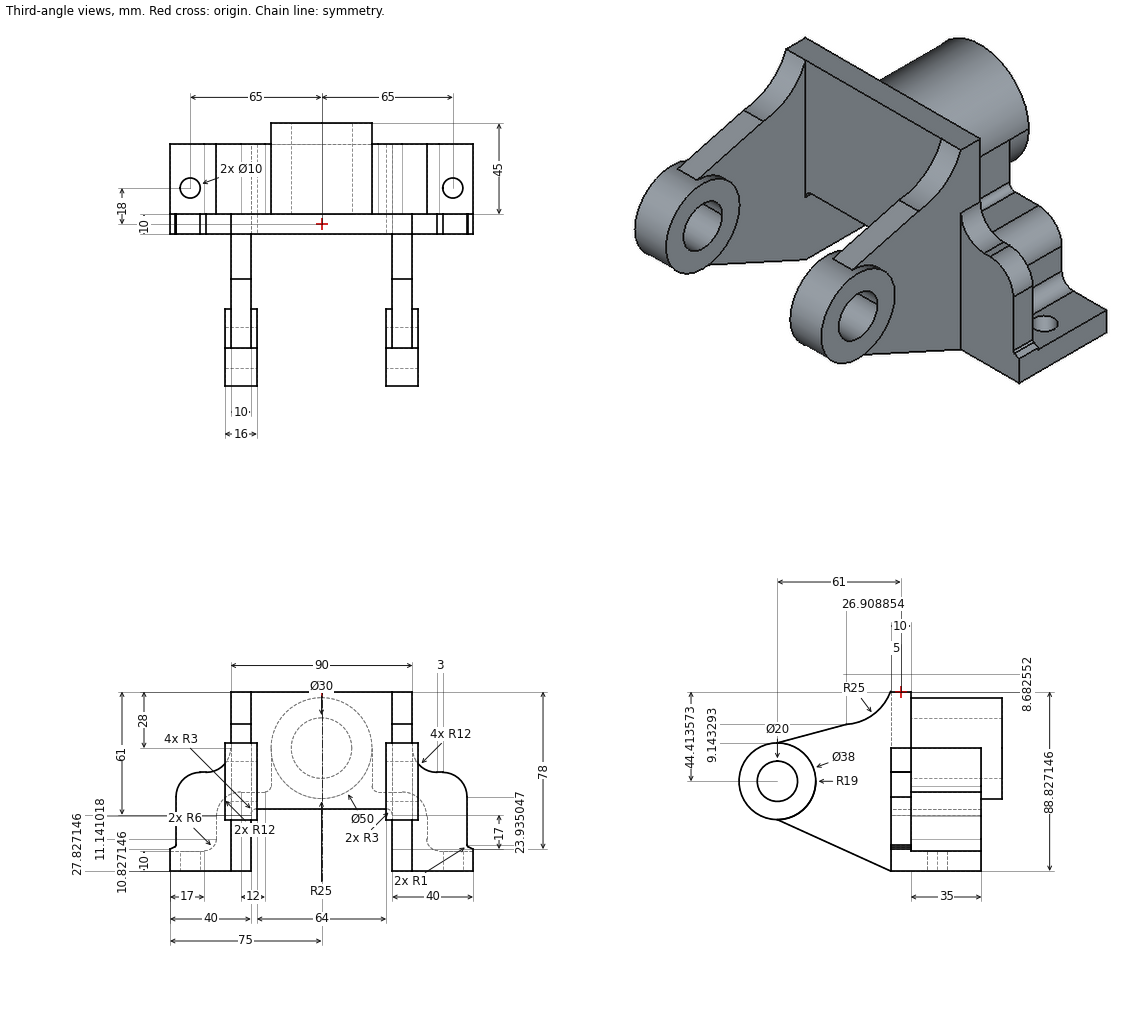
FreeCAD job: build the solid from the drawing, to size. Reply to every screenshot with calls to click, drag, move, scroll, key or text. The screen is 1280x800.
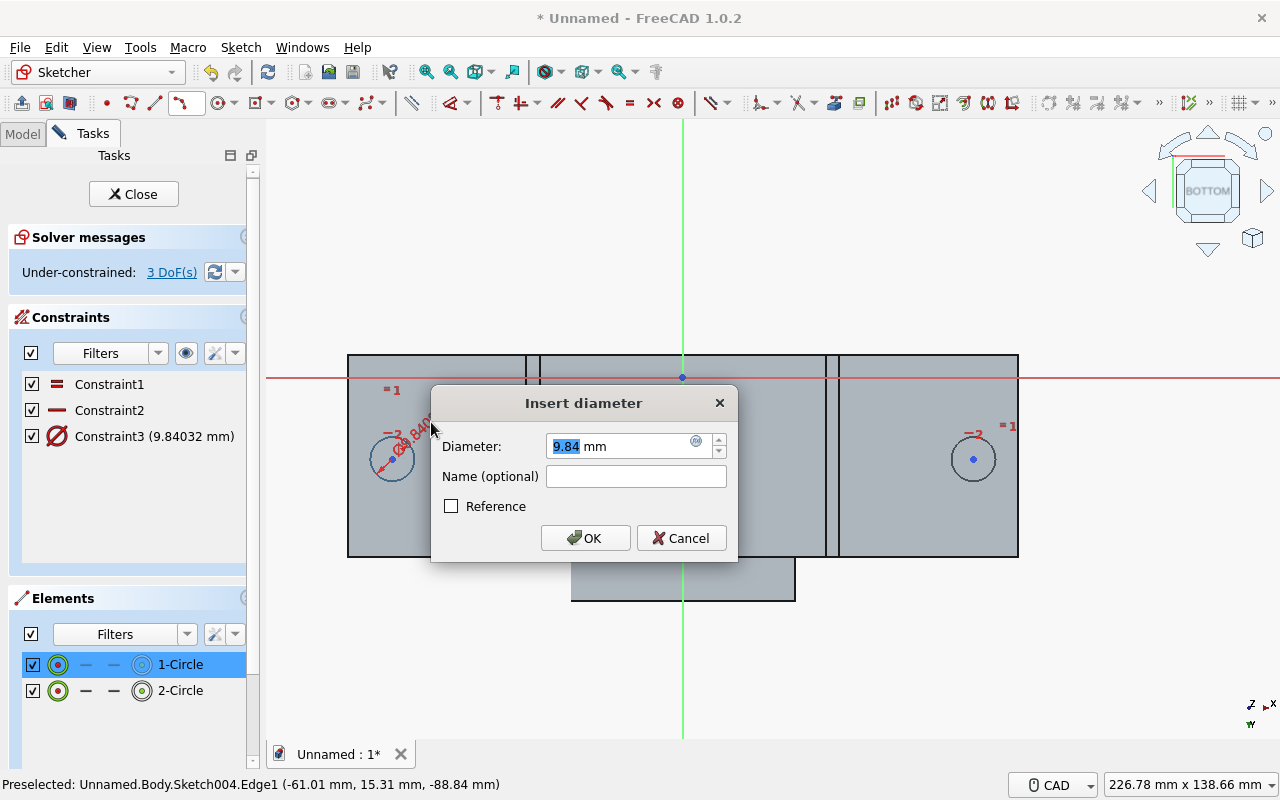
text(10)
key(Return)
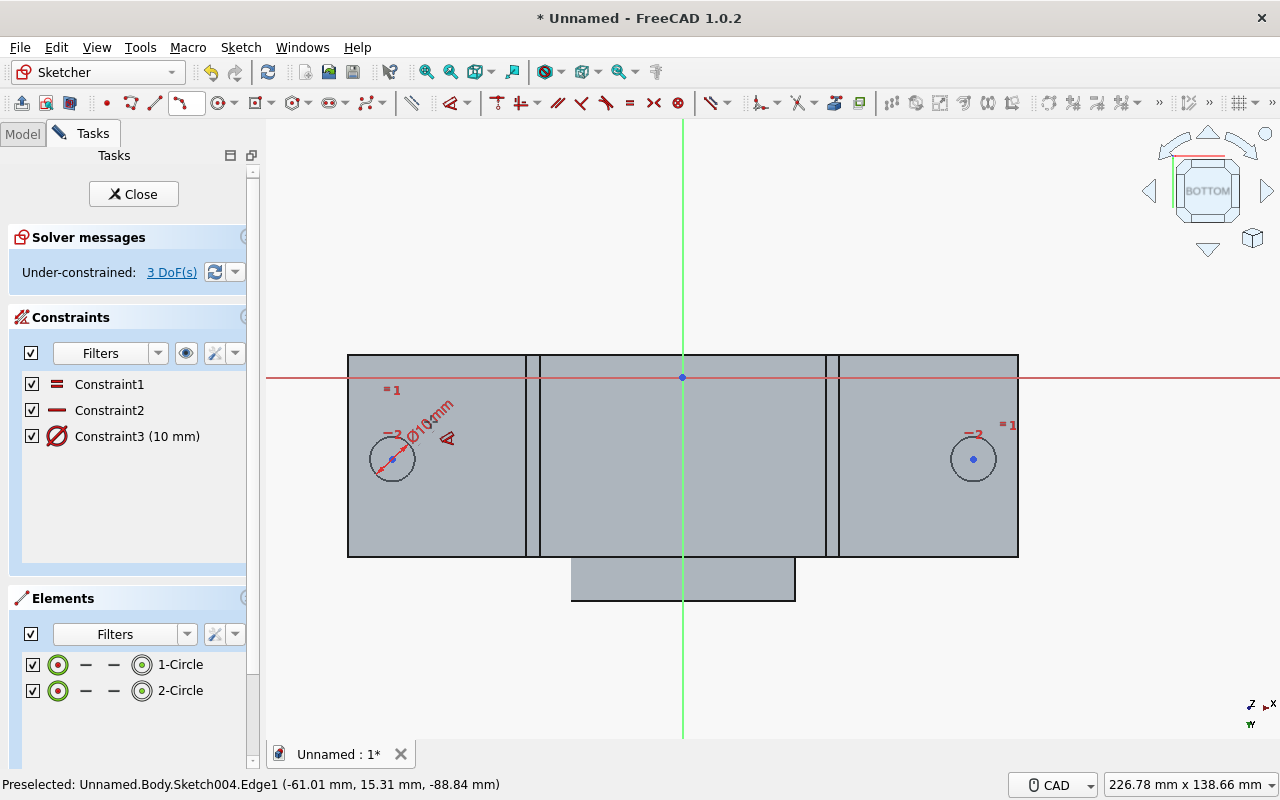
click(392, 459)
click(538, 344)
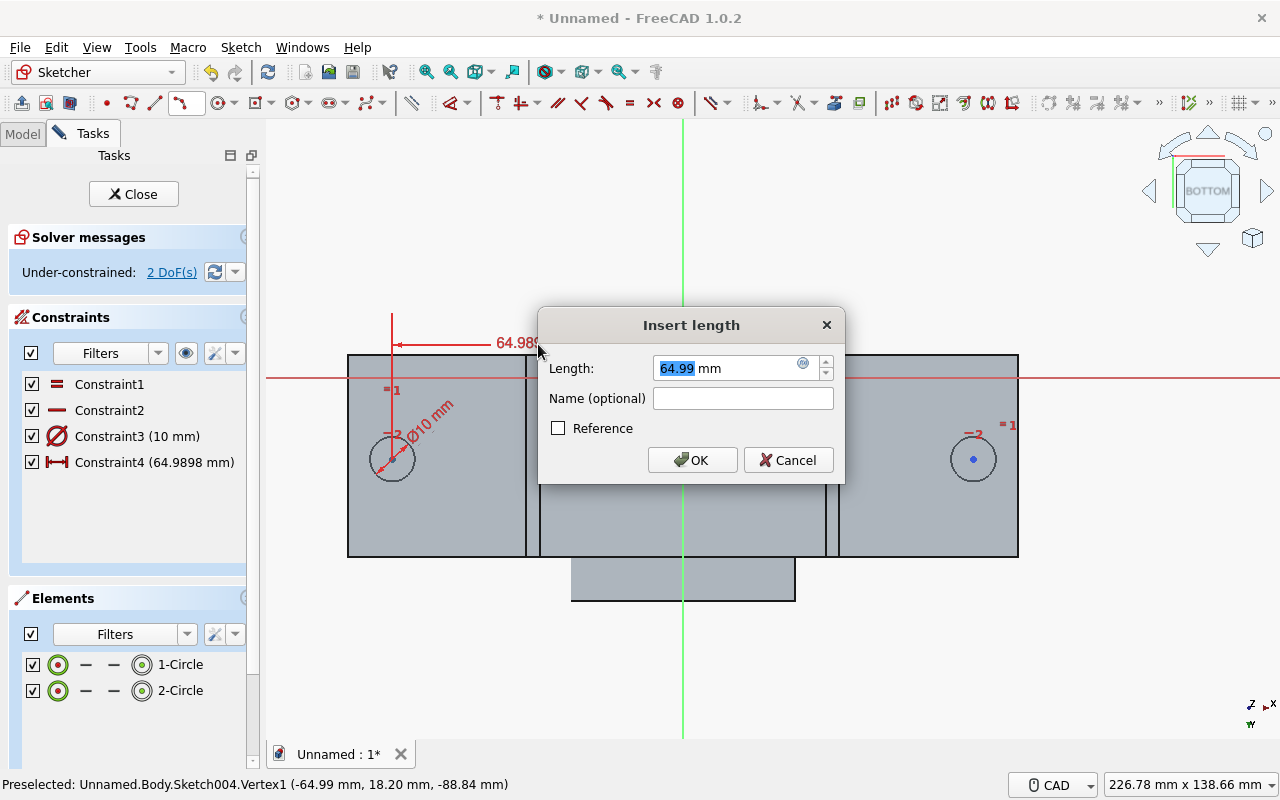
text(65)
key(Return)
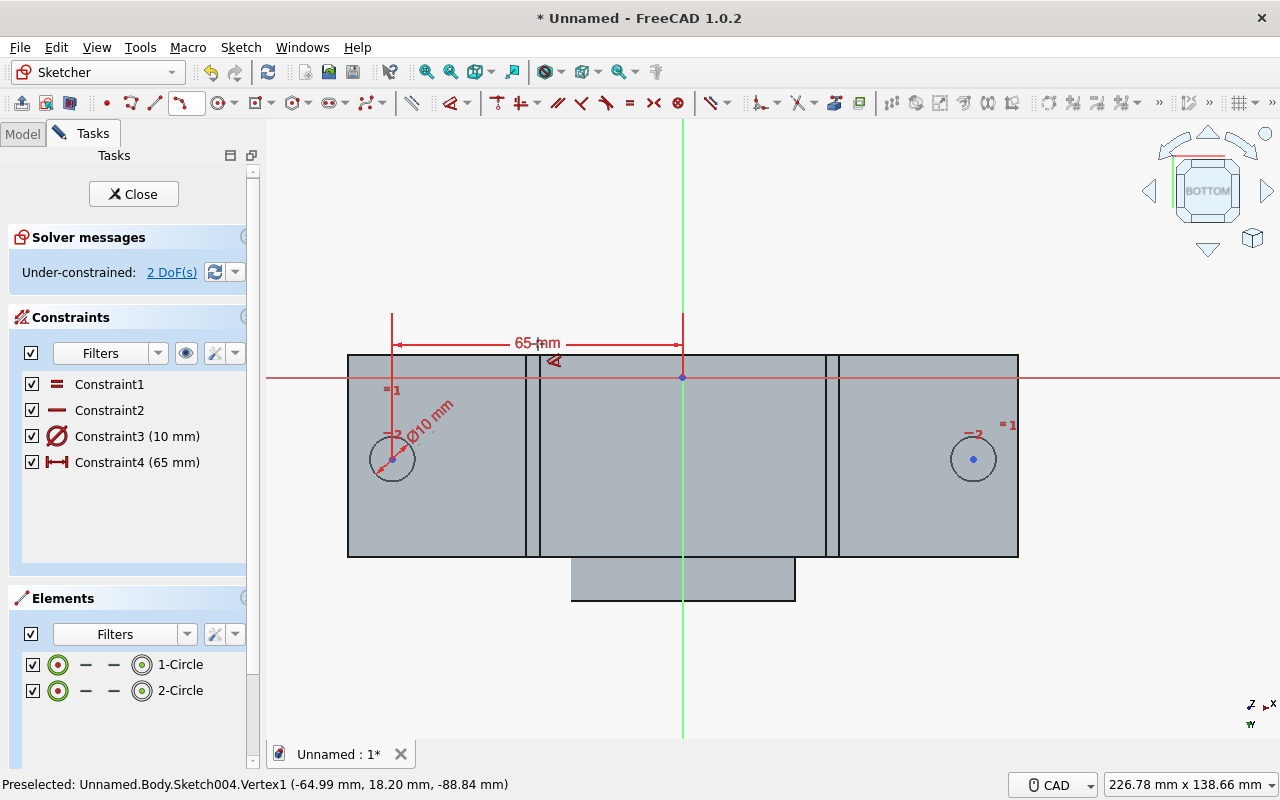
click(392, 459)
click(358, 418)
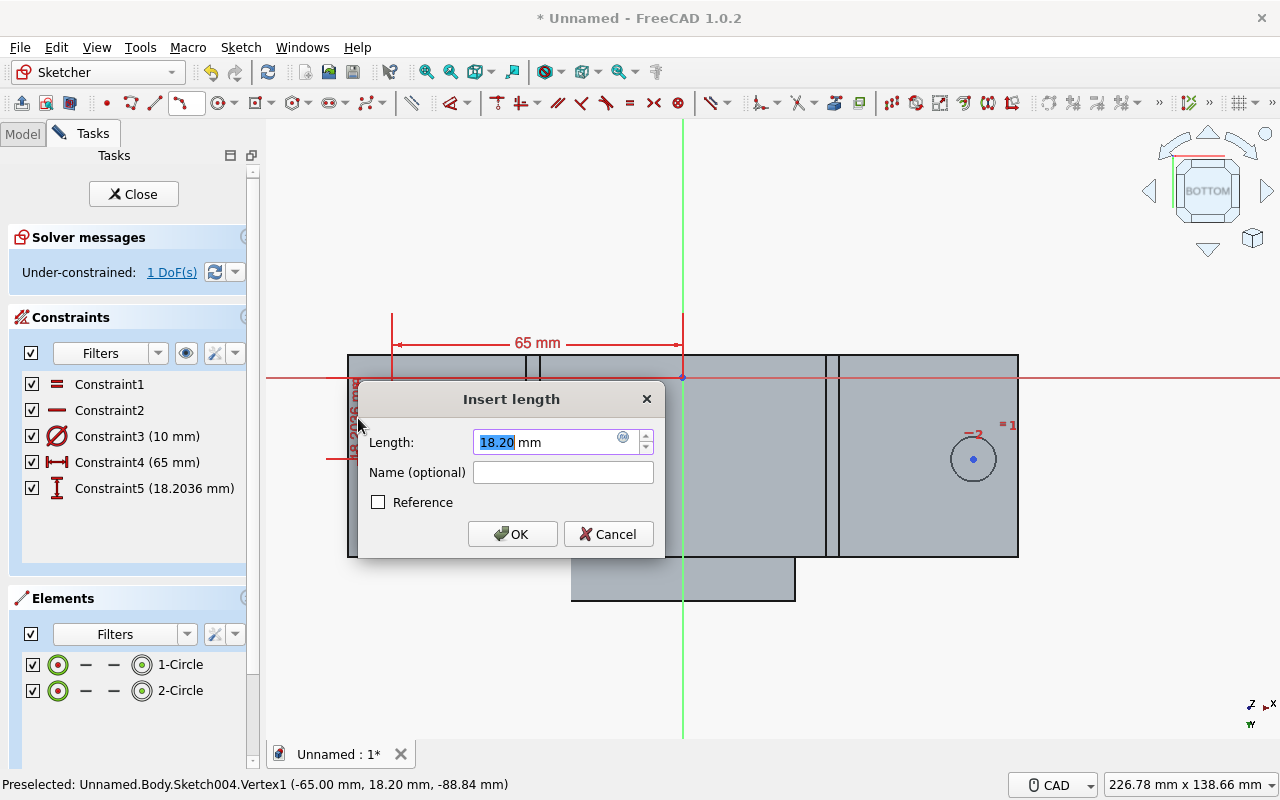
text(18)
key(Return)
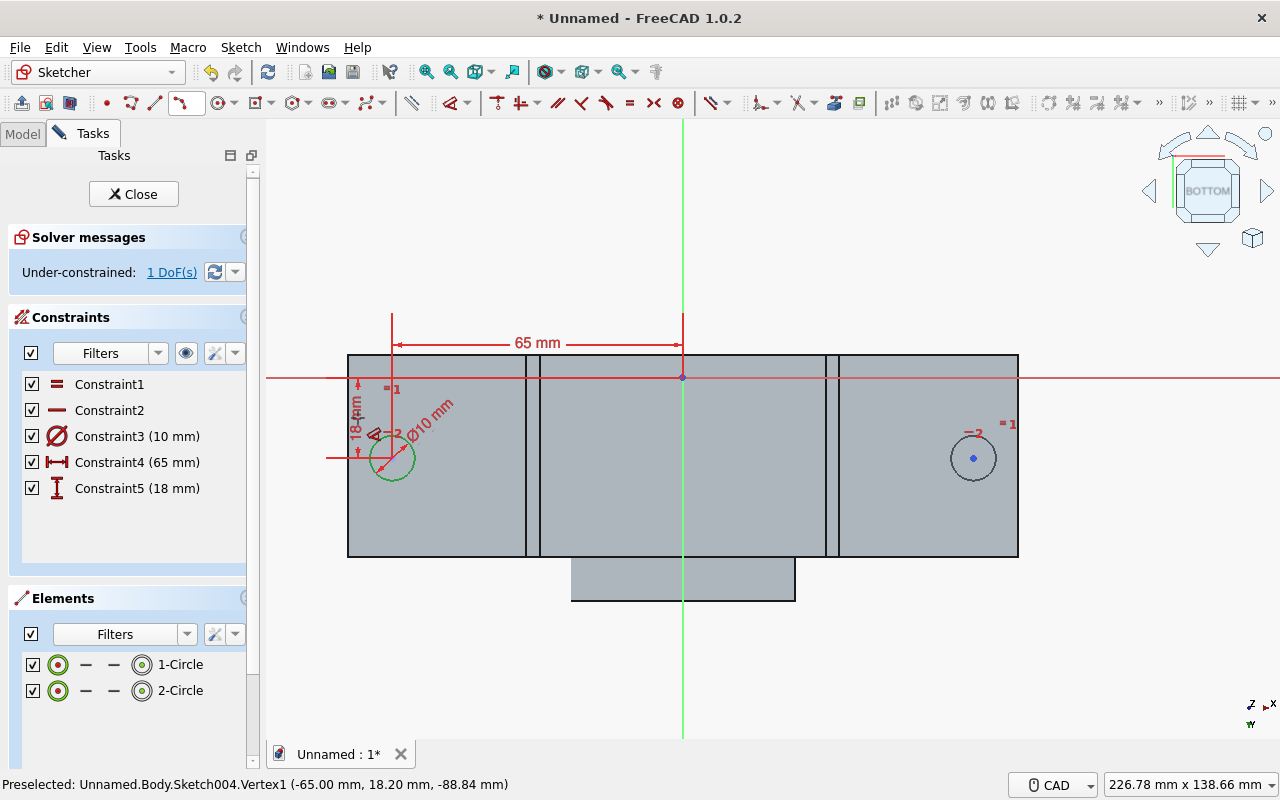
click(974, 458)
click(828, 344)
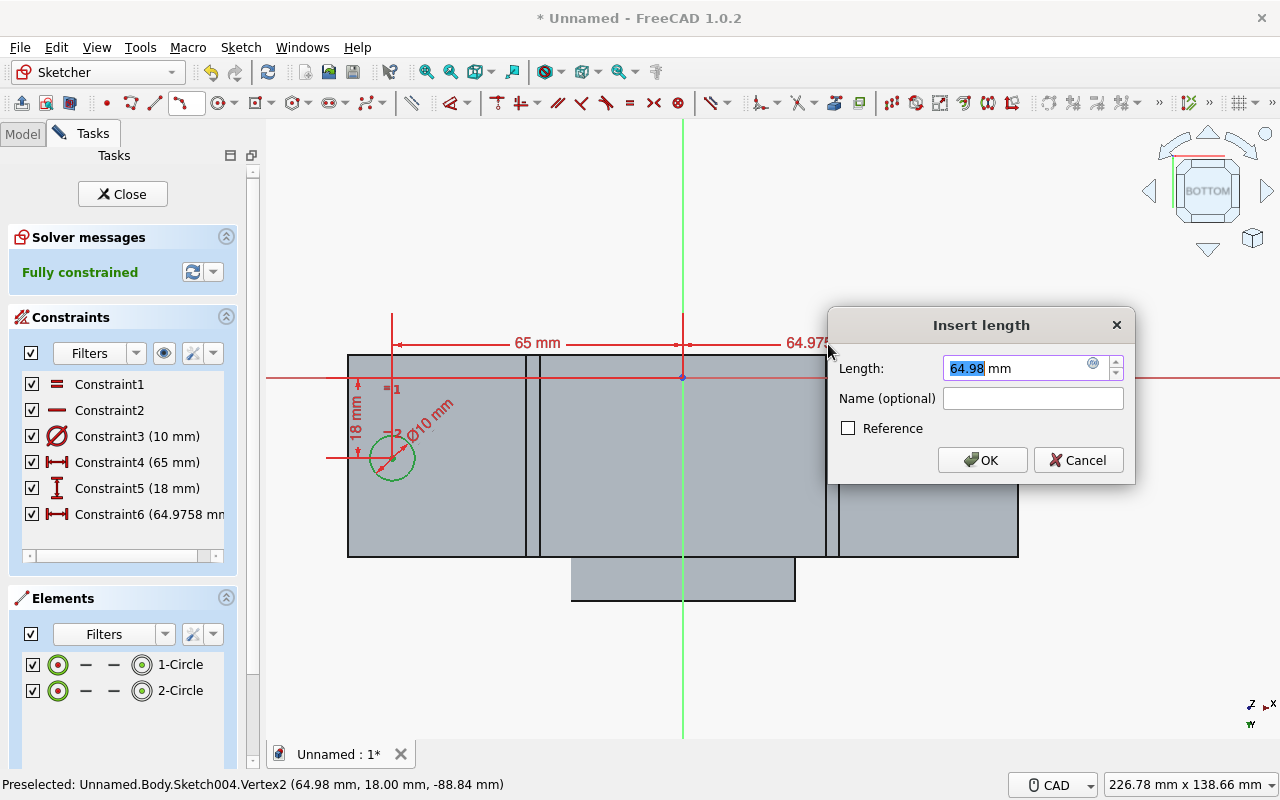
text(65)
key(Return)
key(Escape)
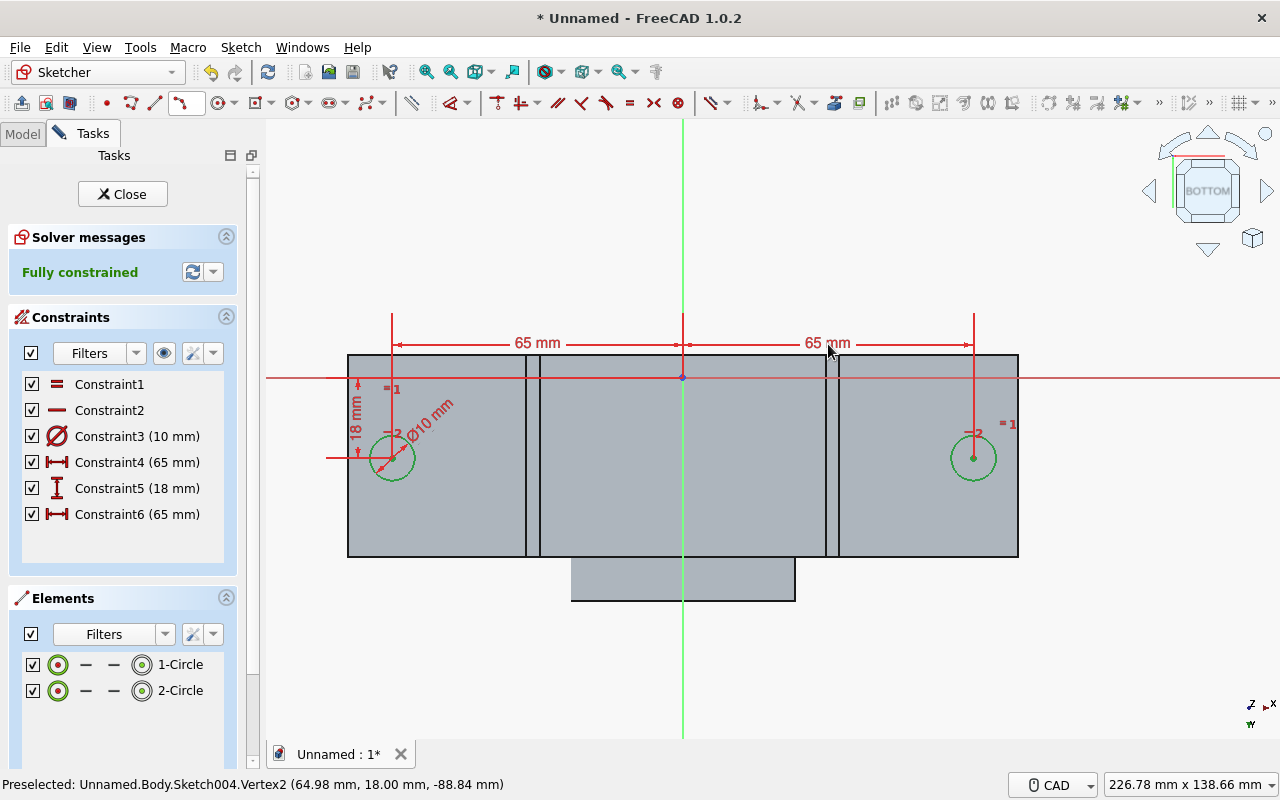
click(123, 194)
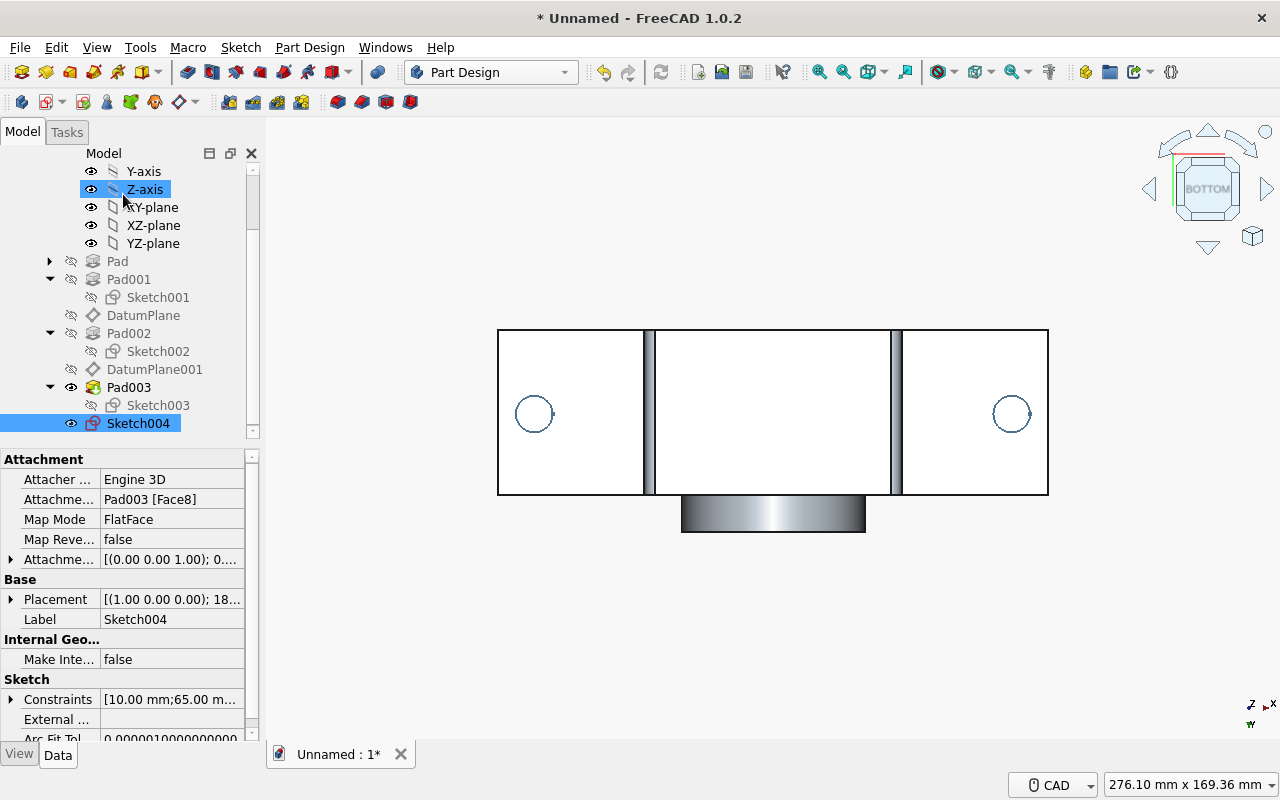
click(188, 72)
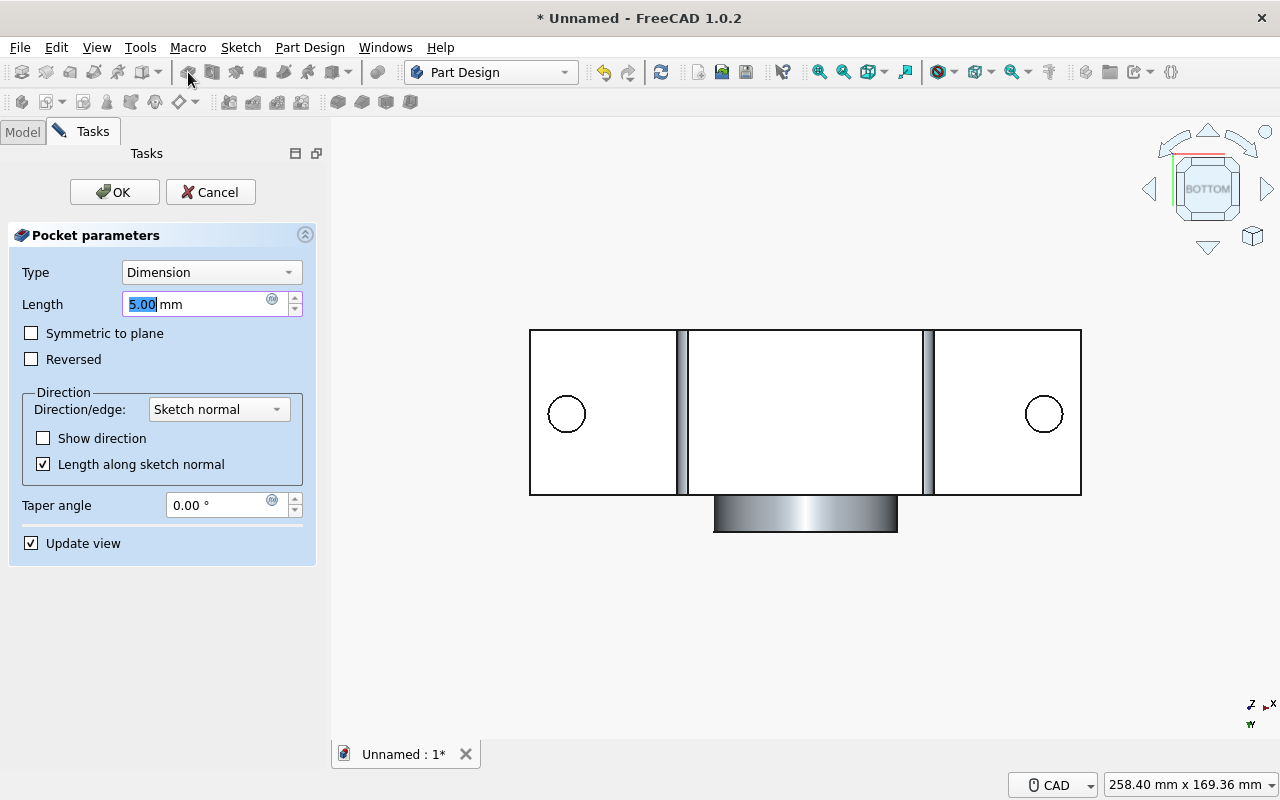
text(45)
key(Tab)